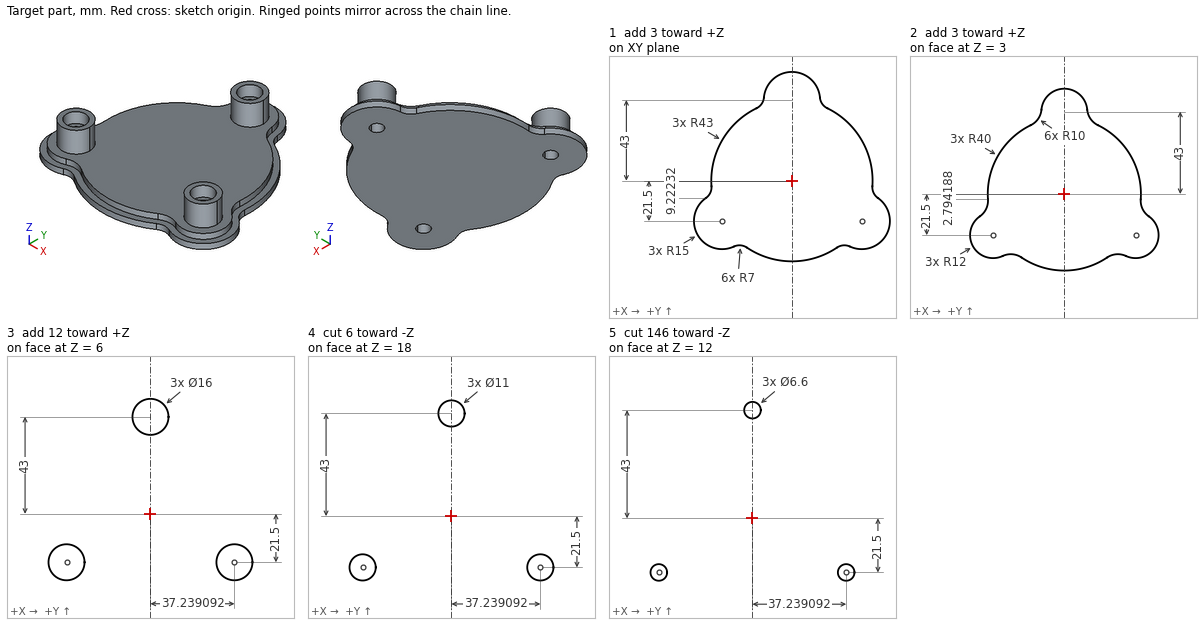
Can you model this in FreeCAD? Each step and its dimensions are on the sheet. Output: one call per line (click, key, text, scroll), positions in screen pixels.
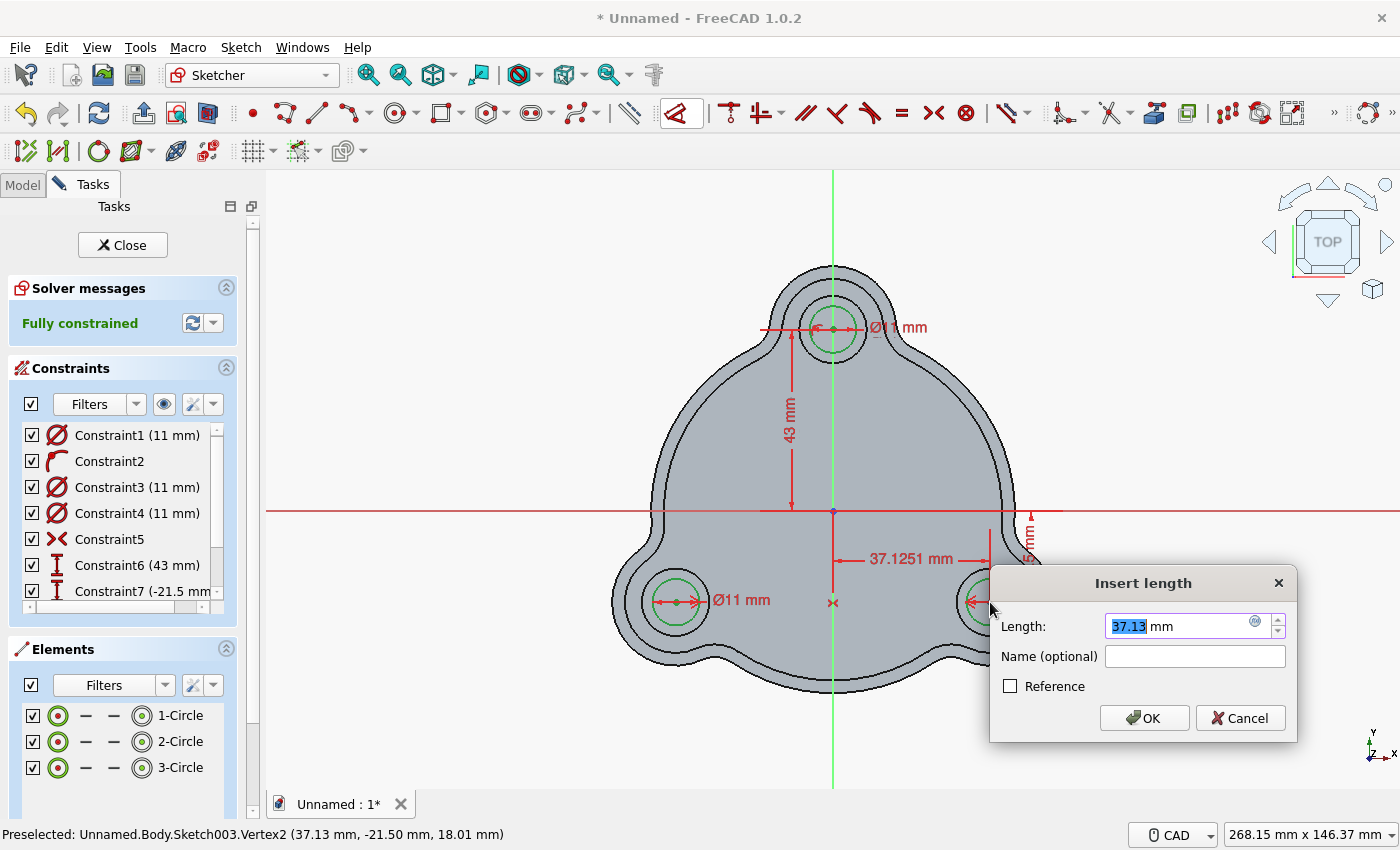
text(37.239092)
key(Return)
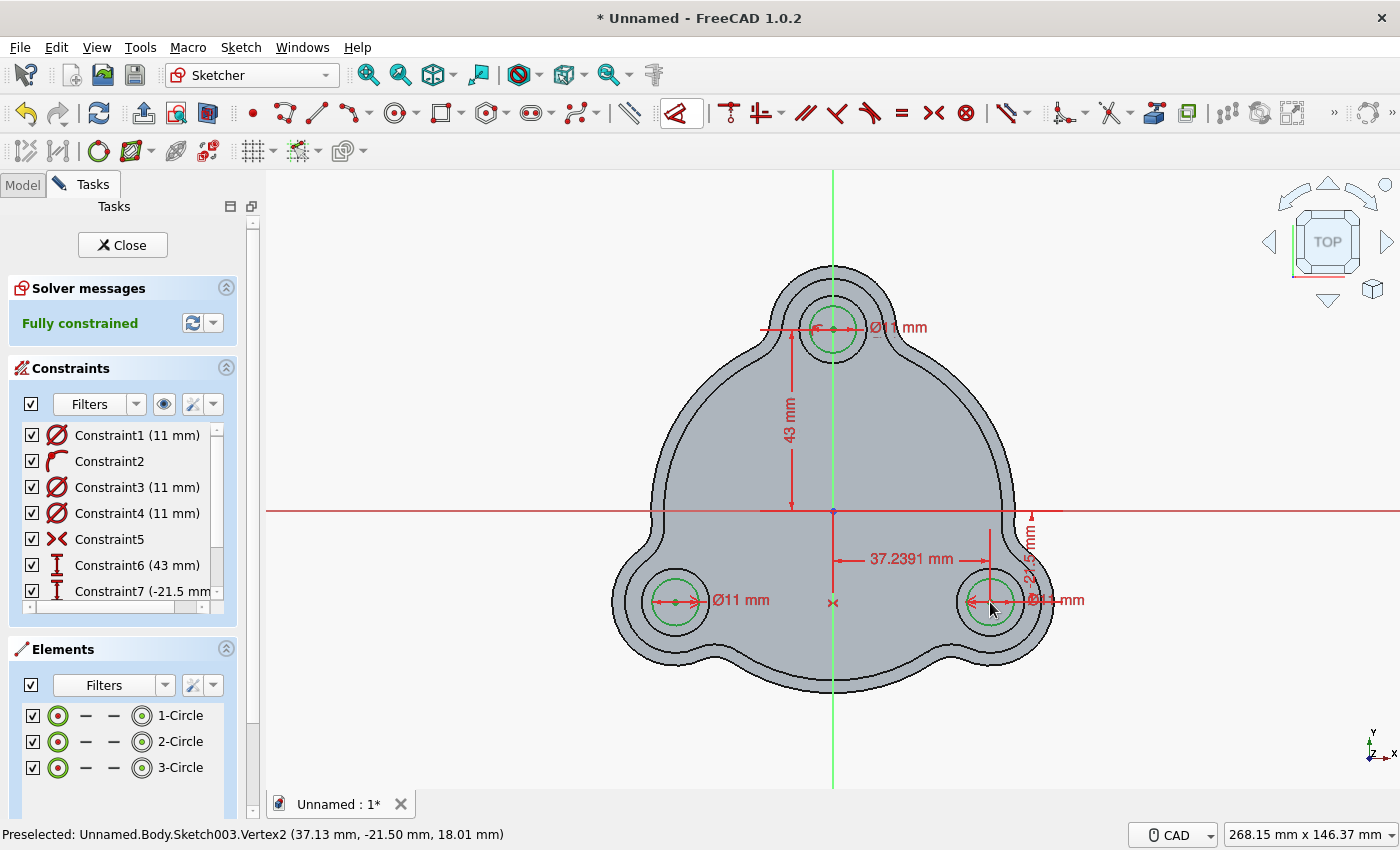
click(123, 245)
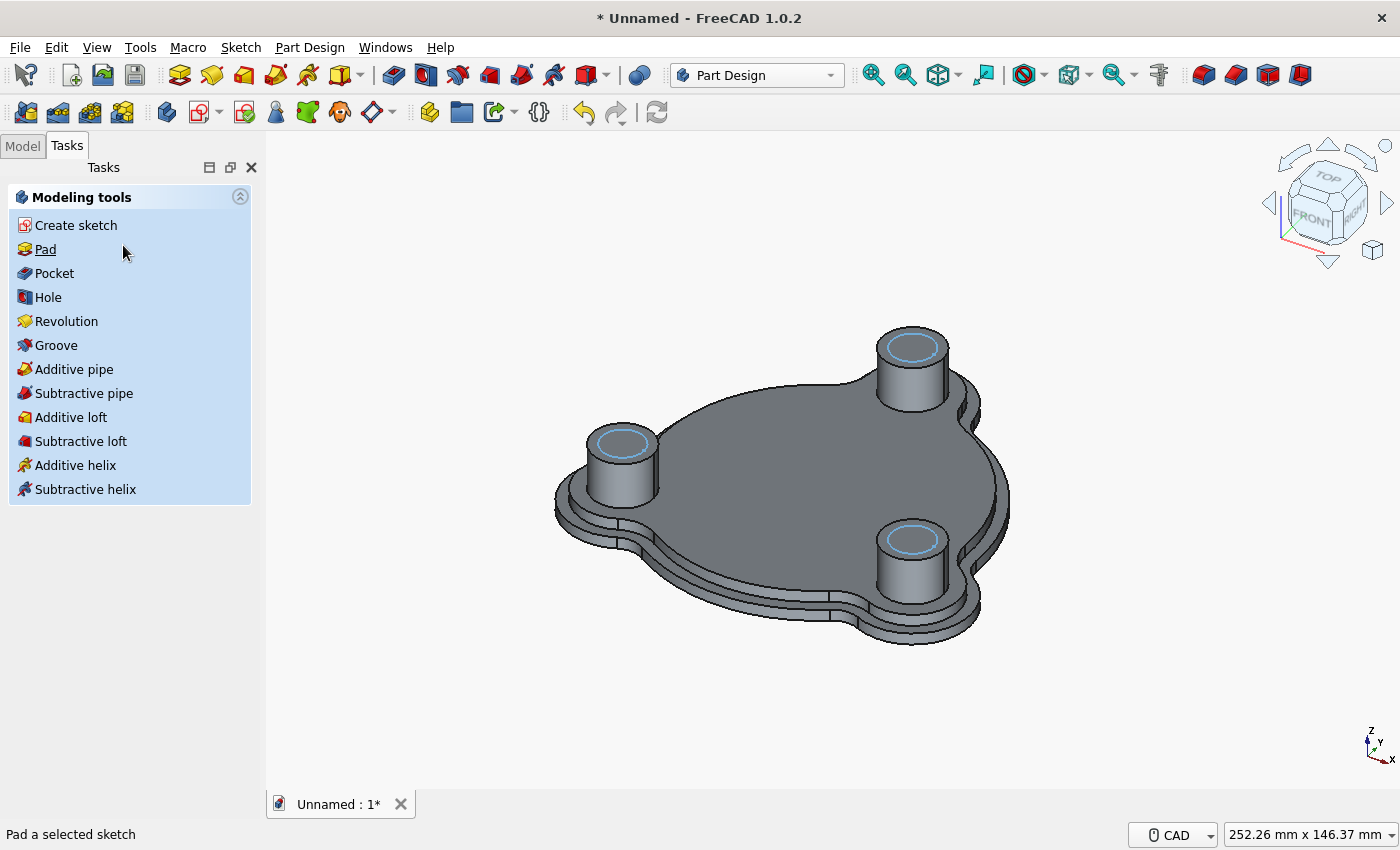
click(394, 76)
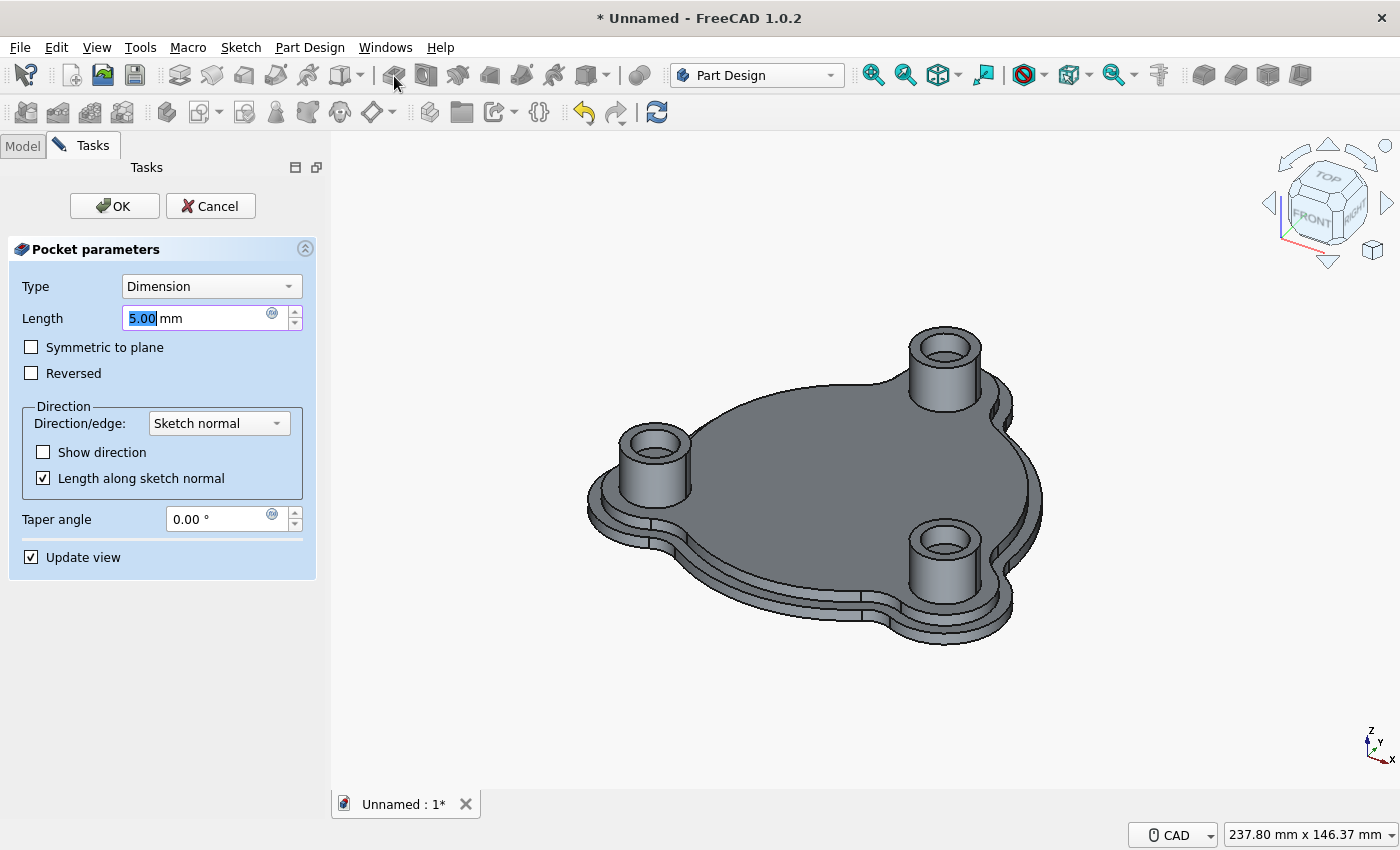
text(6)
key(Tab)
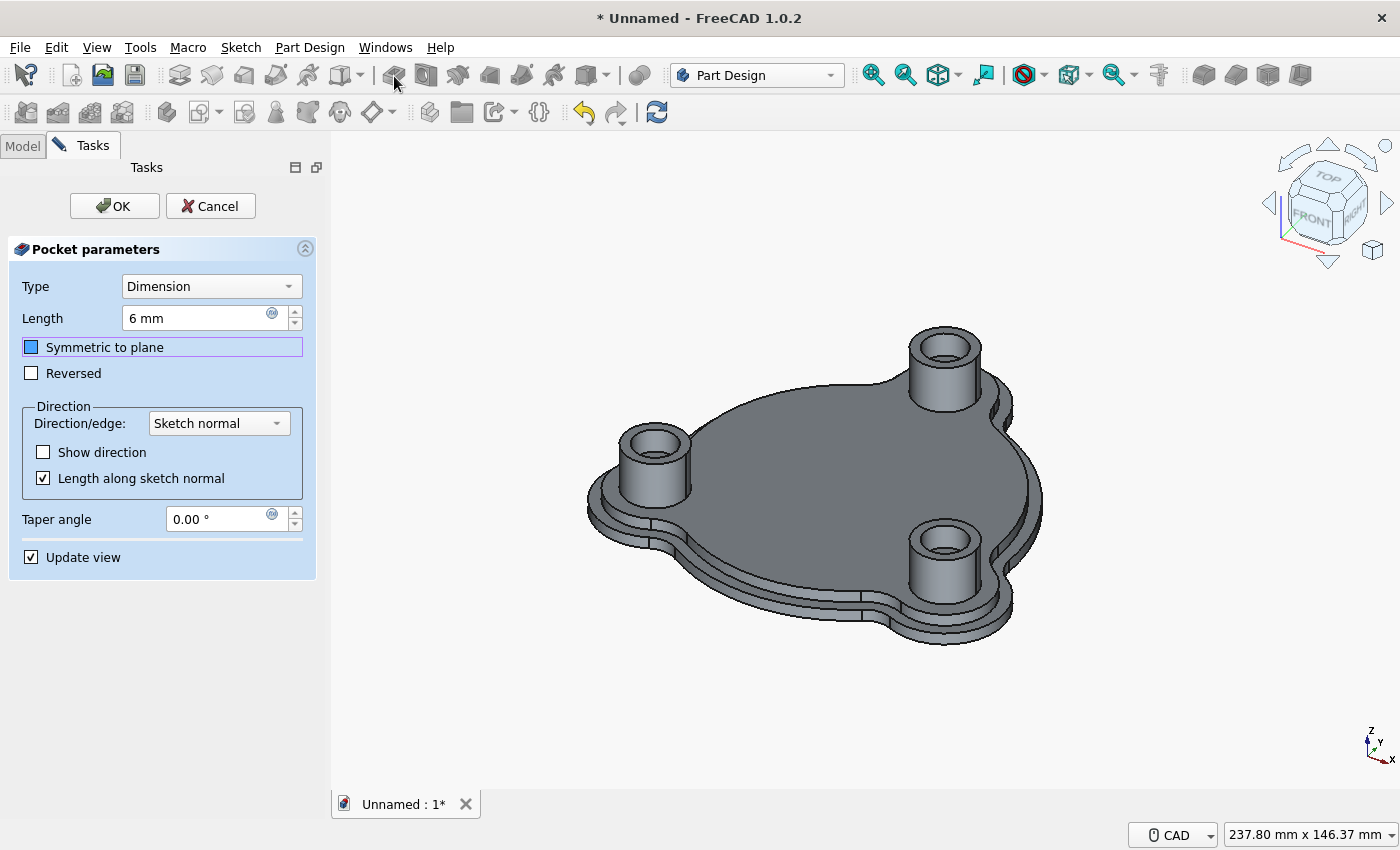
click(115, 206)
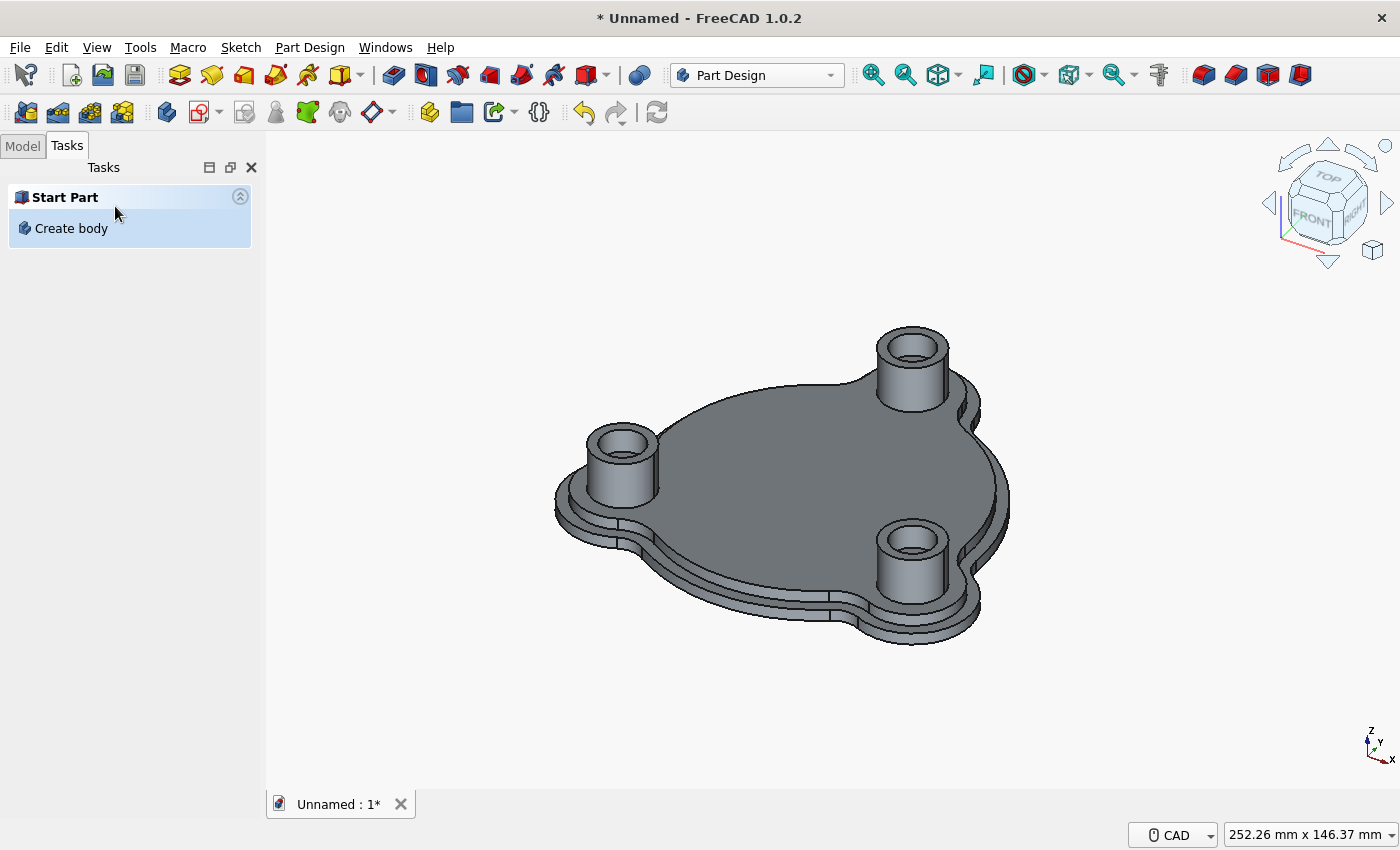
key(0)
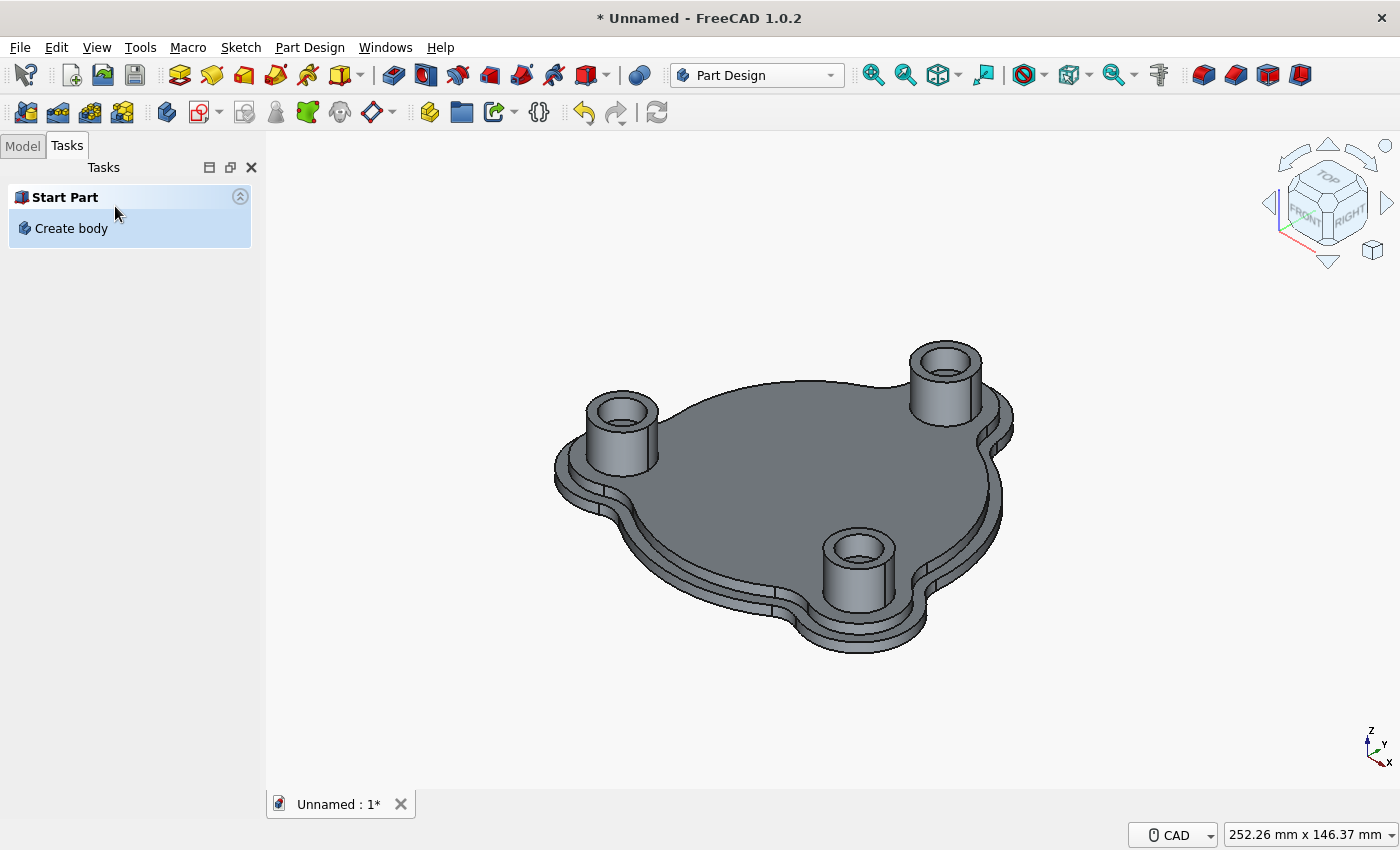
key(2)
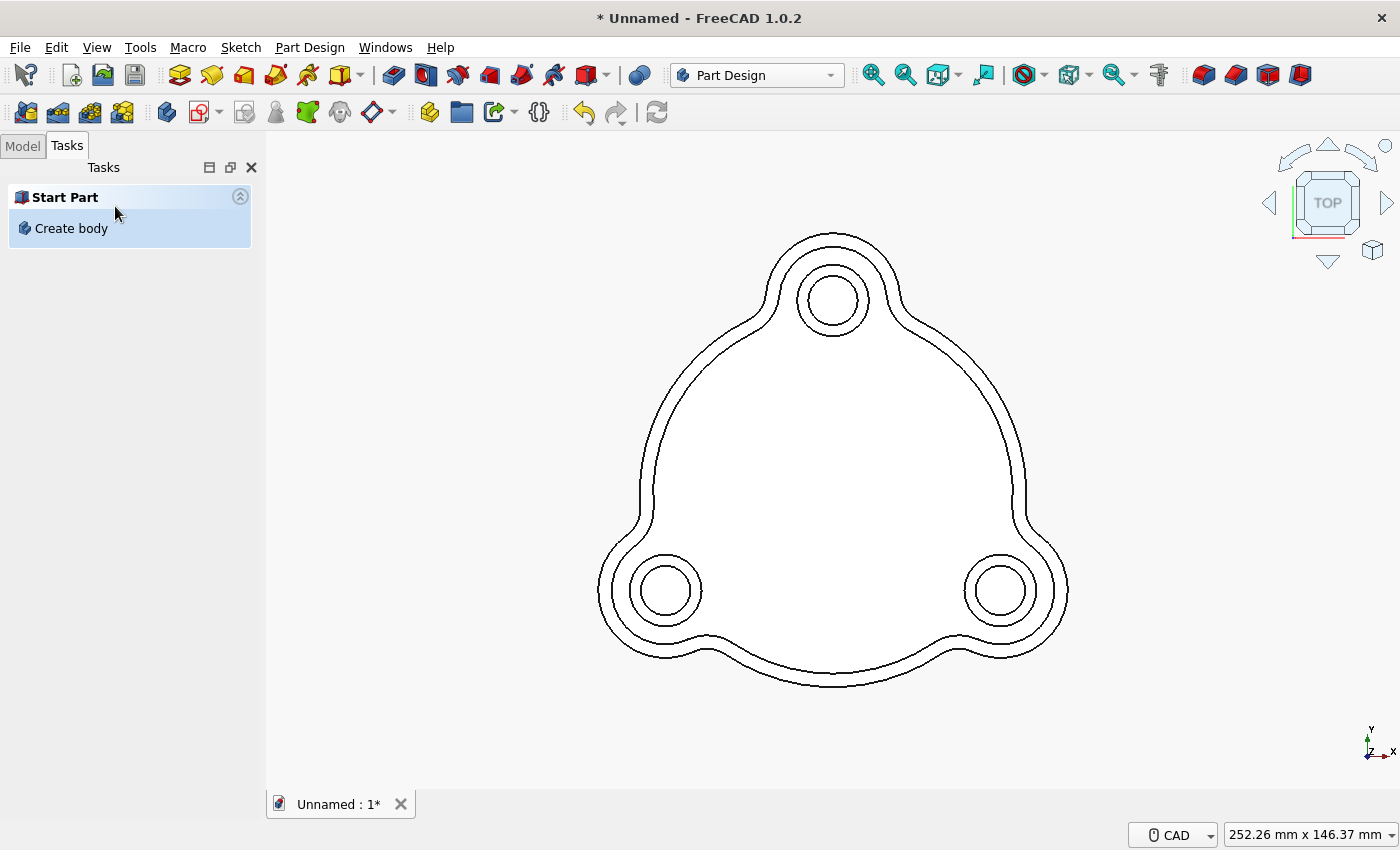
click(833, 300)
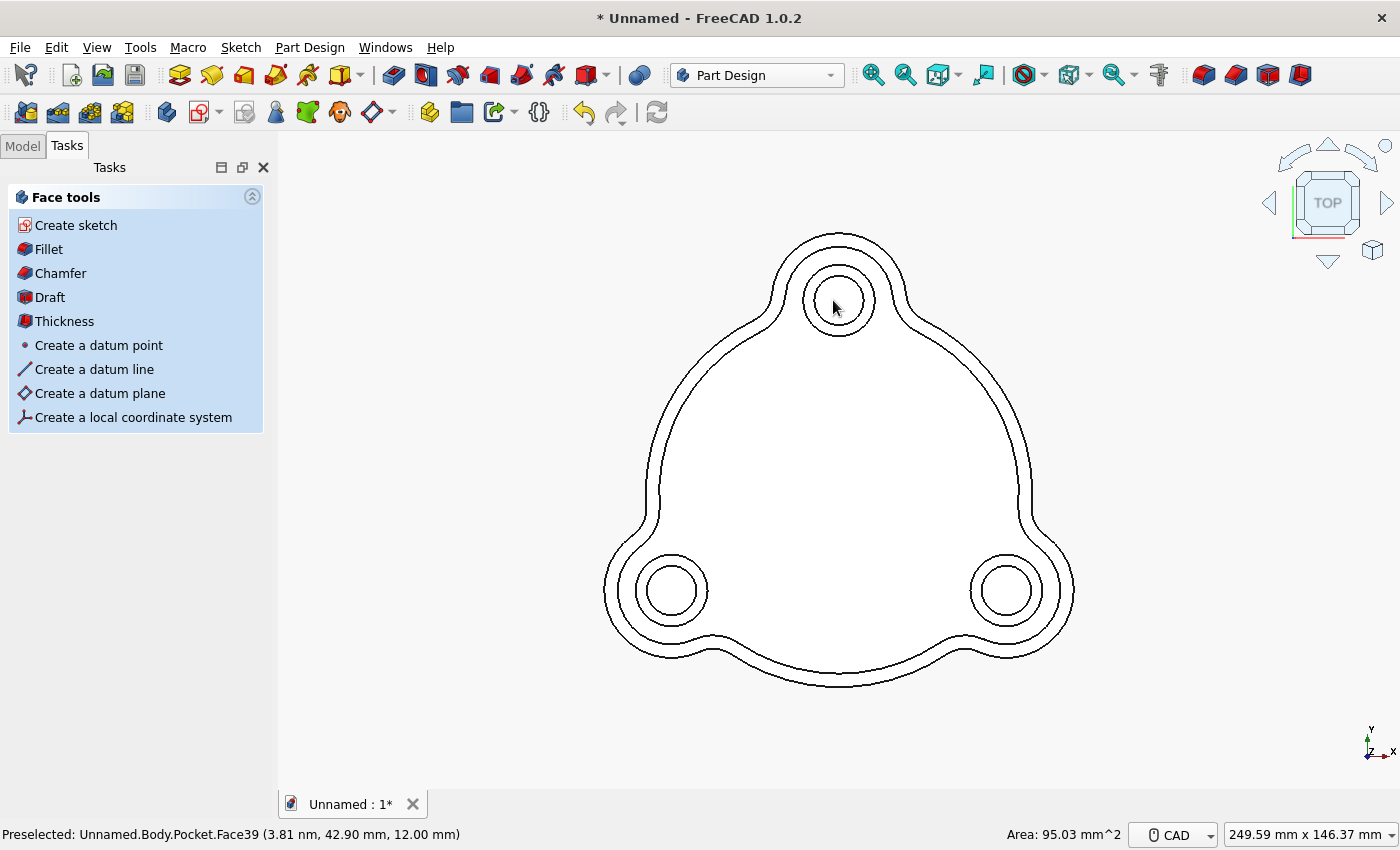
click(200, 112)